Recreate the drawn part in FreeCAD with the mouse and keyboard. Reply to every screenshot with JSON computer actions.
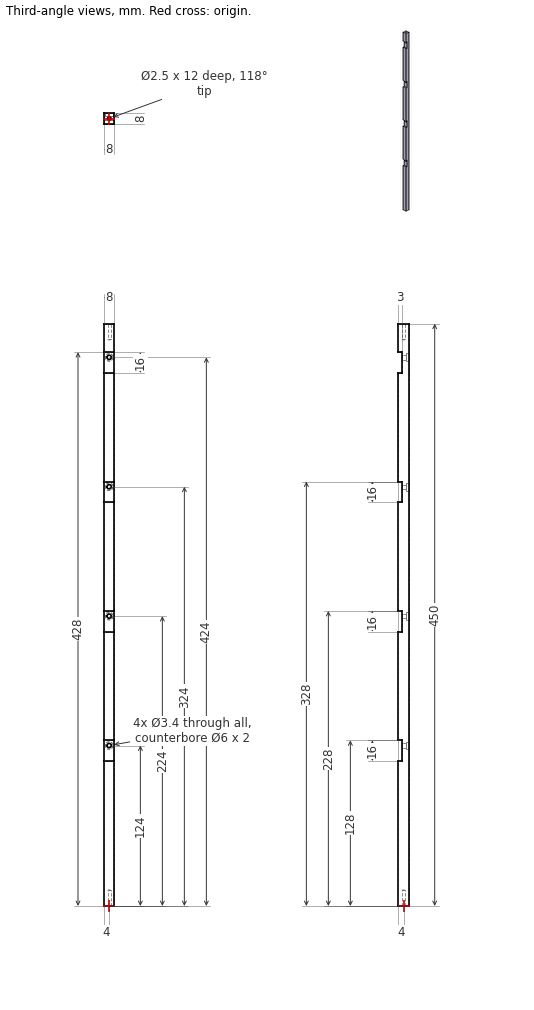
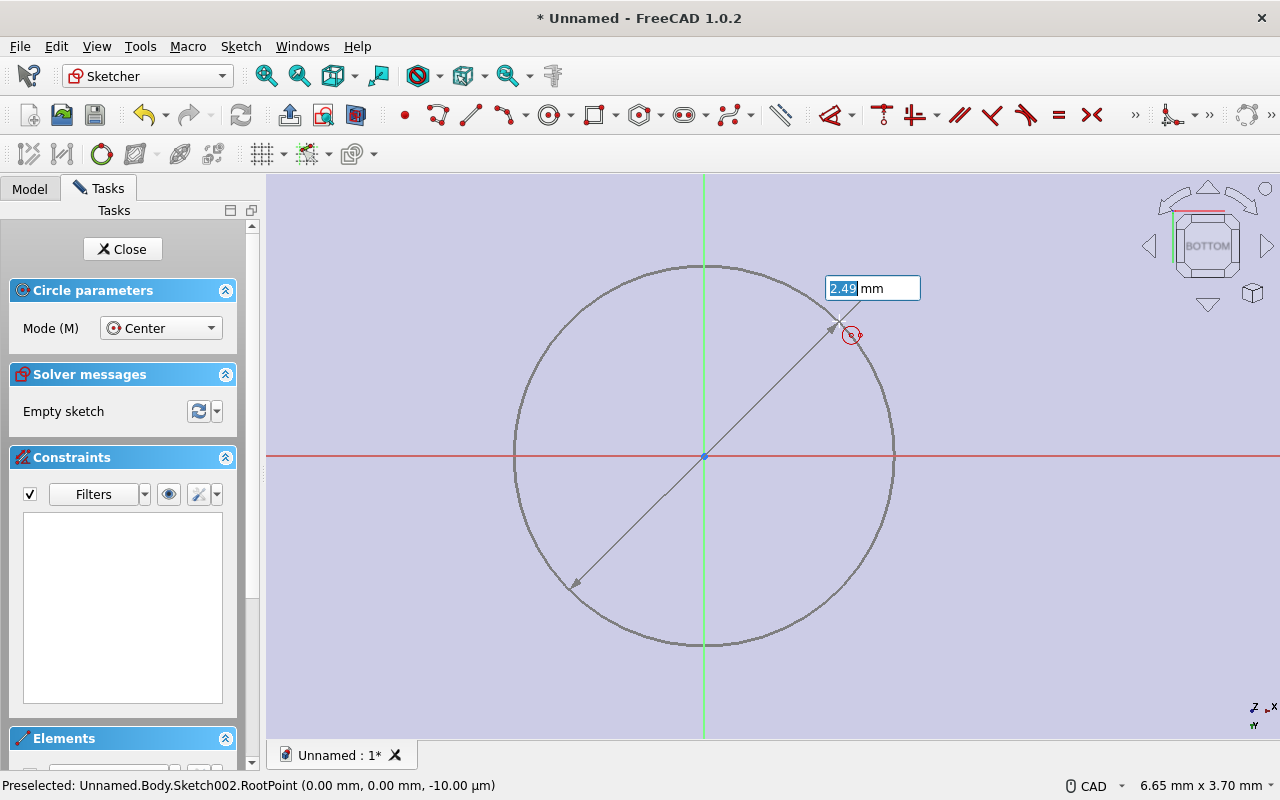
{"action": "type", "text": "2.5"}
{"action": "key", "text": "Return"}
{"action": "key", "text": "Escape"}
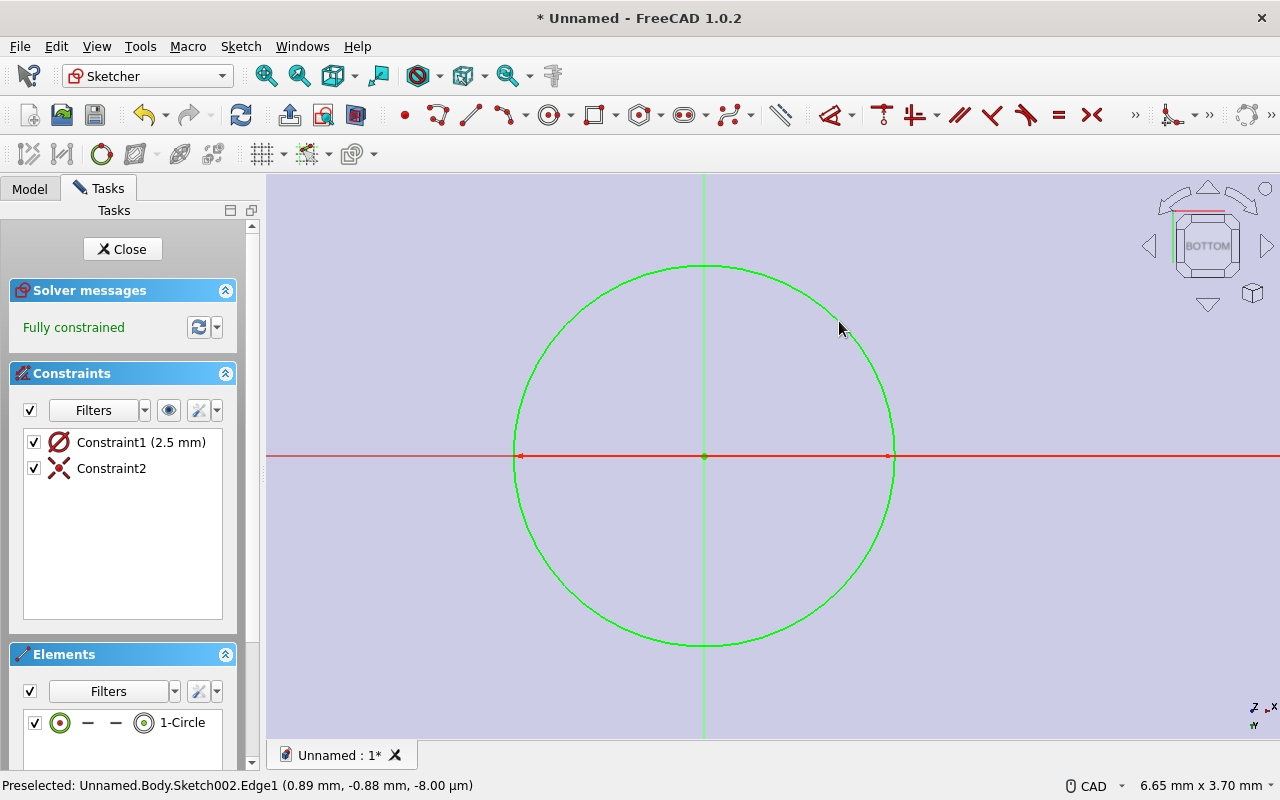
{"action": "left_click", "coordinate": [123, 249]}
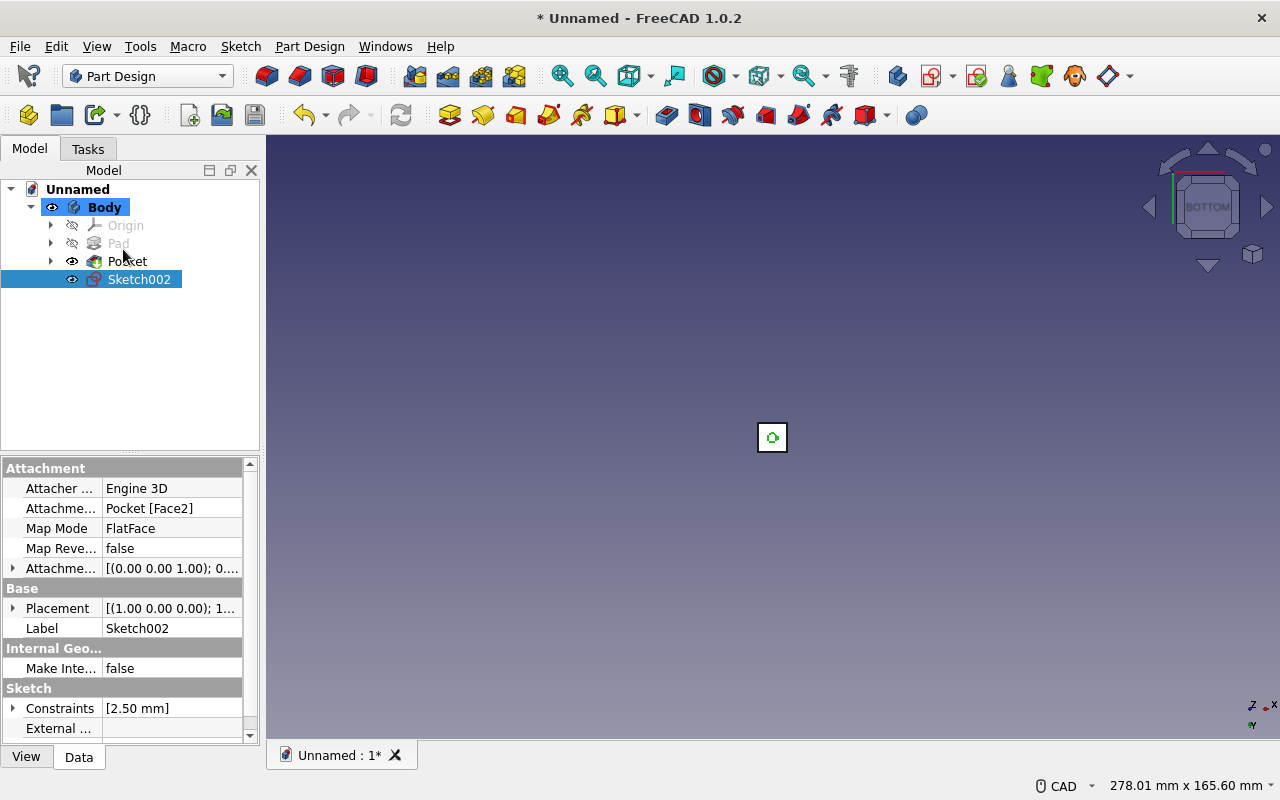
{"action": "left_click", "coordinate": [700, 116]}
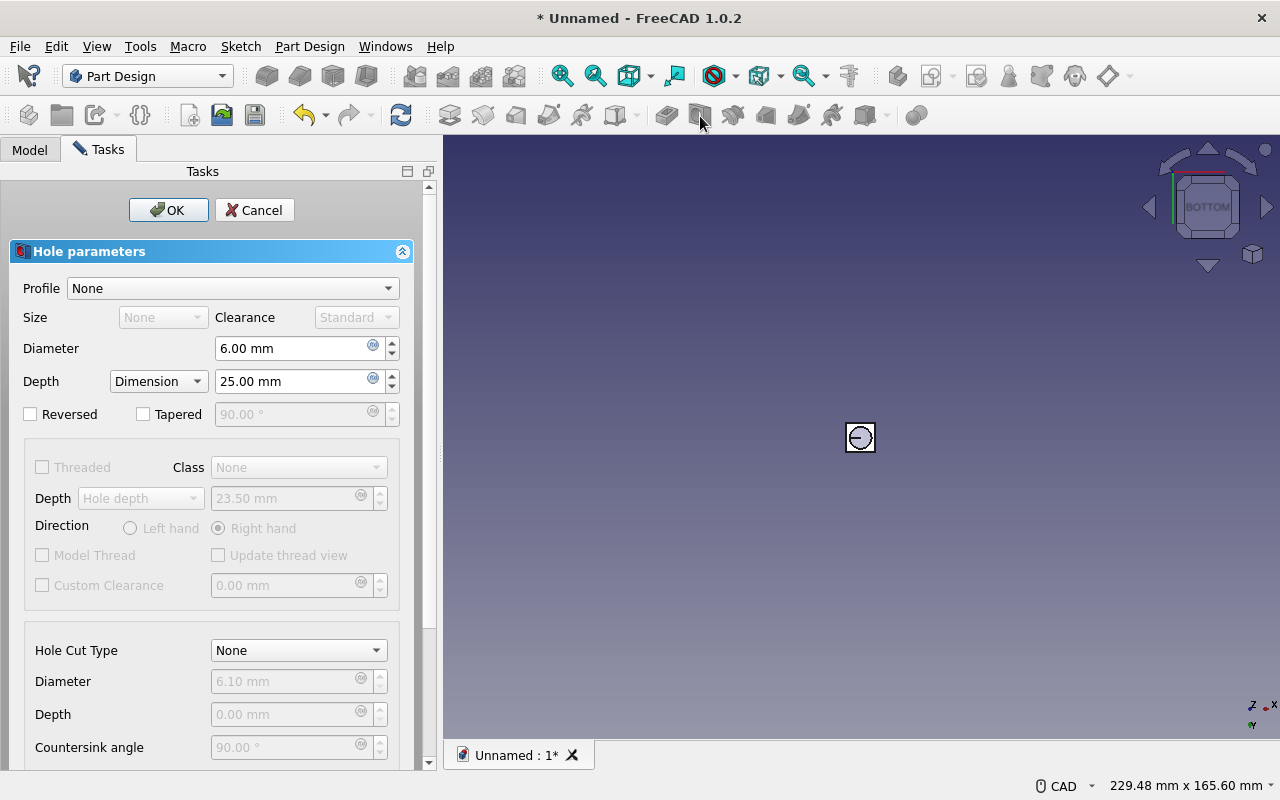
{"action": "triple_click", "coordinate": [300, 348]}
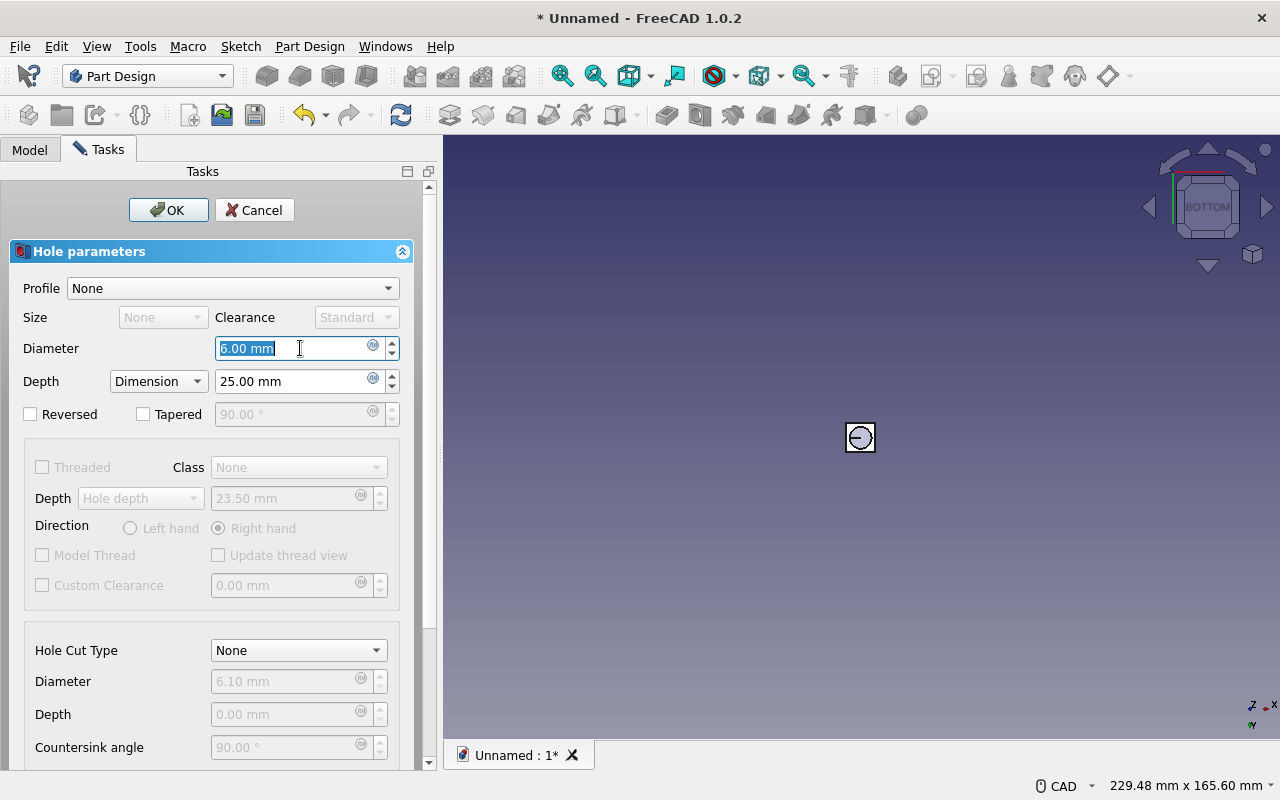
{"action": "type", "text": "2.5"}
{"action": "key", "text": "Tab"}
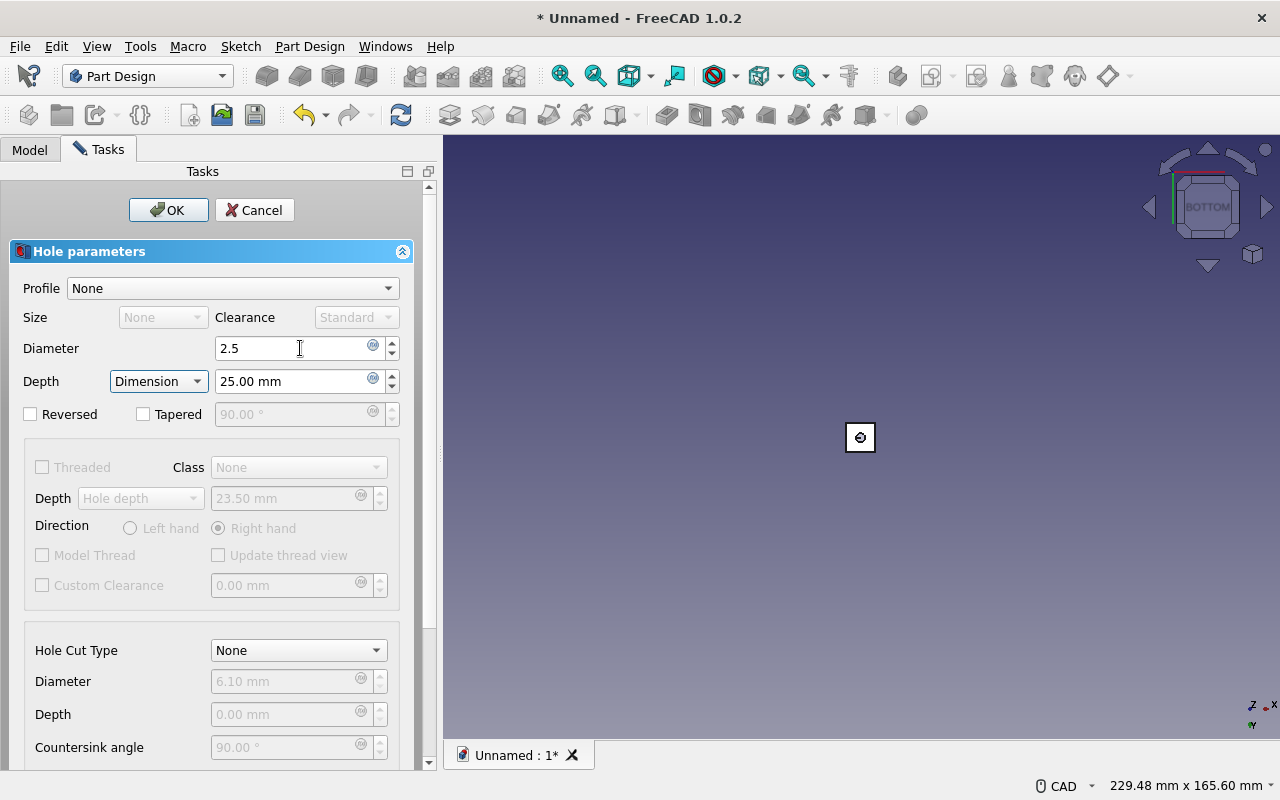
{"action": "triple_click", "coordinate": [300, 382]}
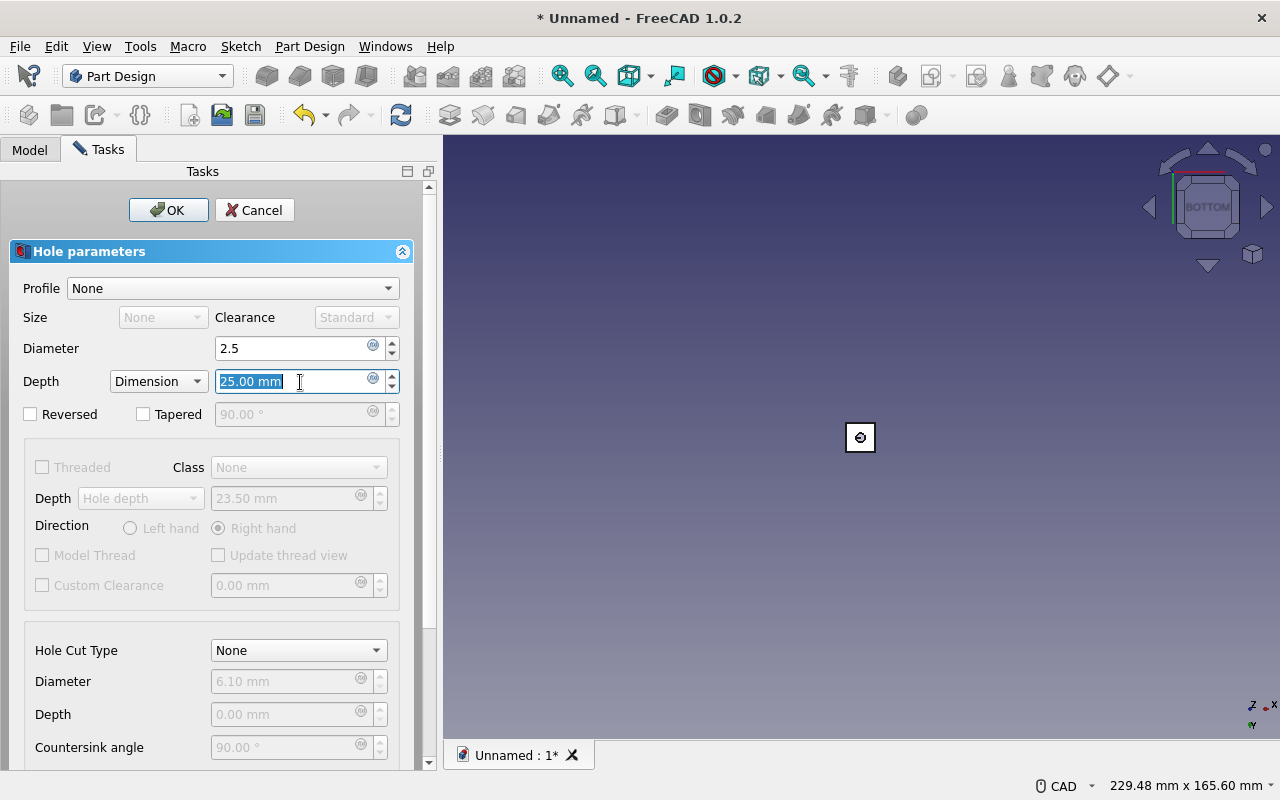
{"action": "type", "text": "12"}
{"action": "key", "text": "Tab"}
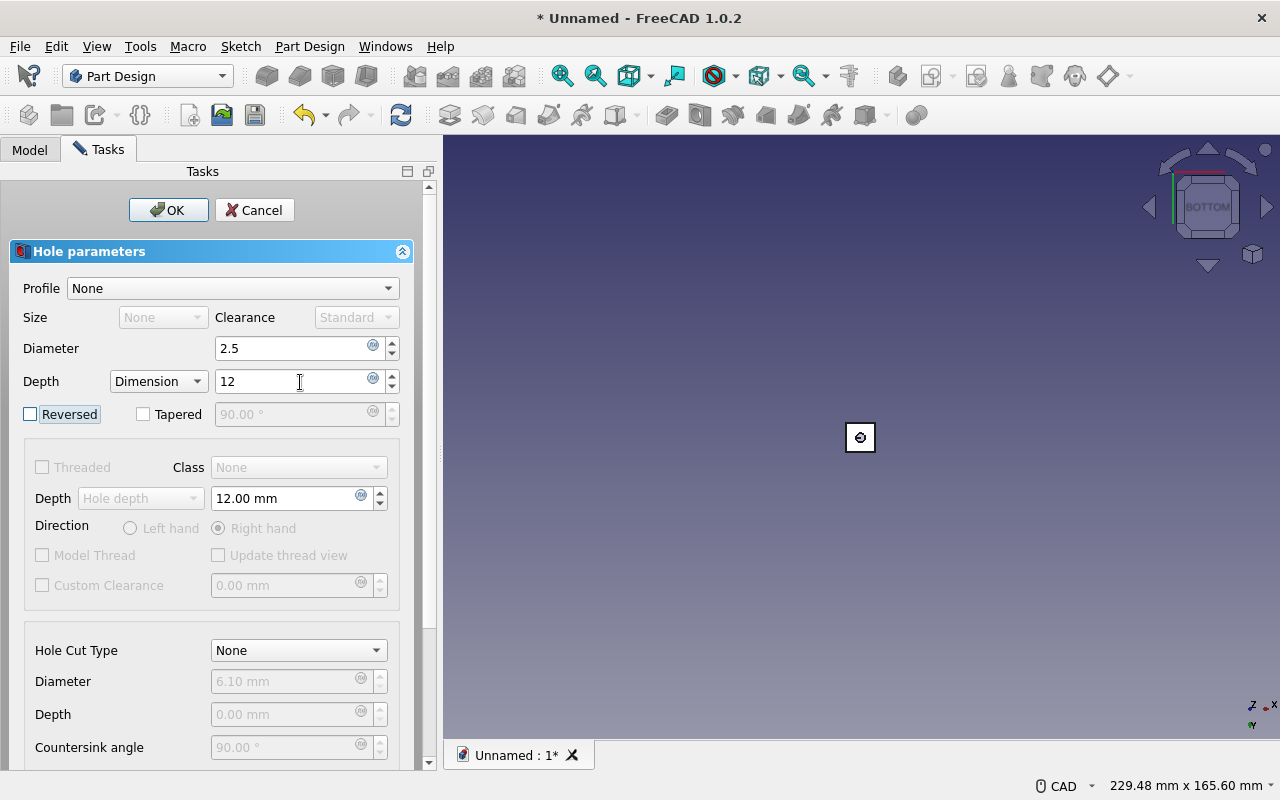
{"action": "left_click", "coordinate": [169, 210]}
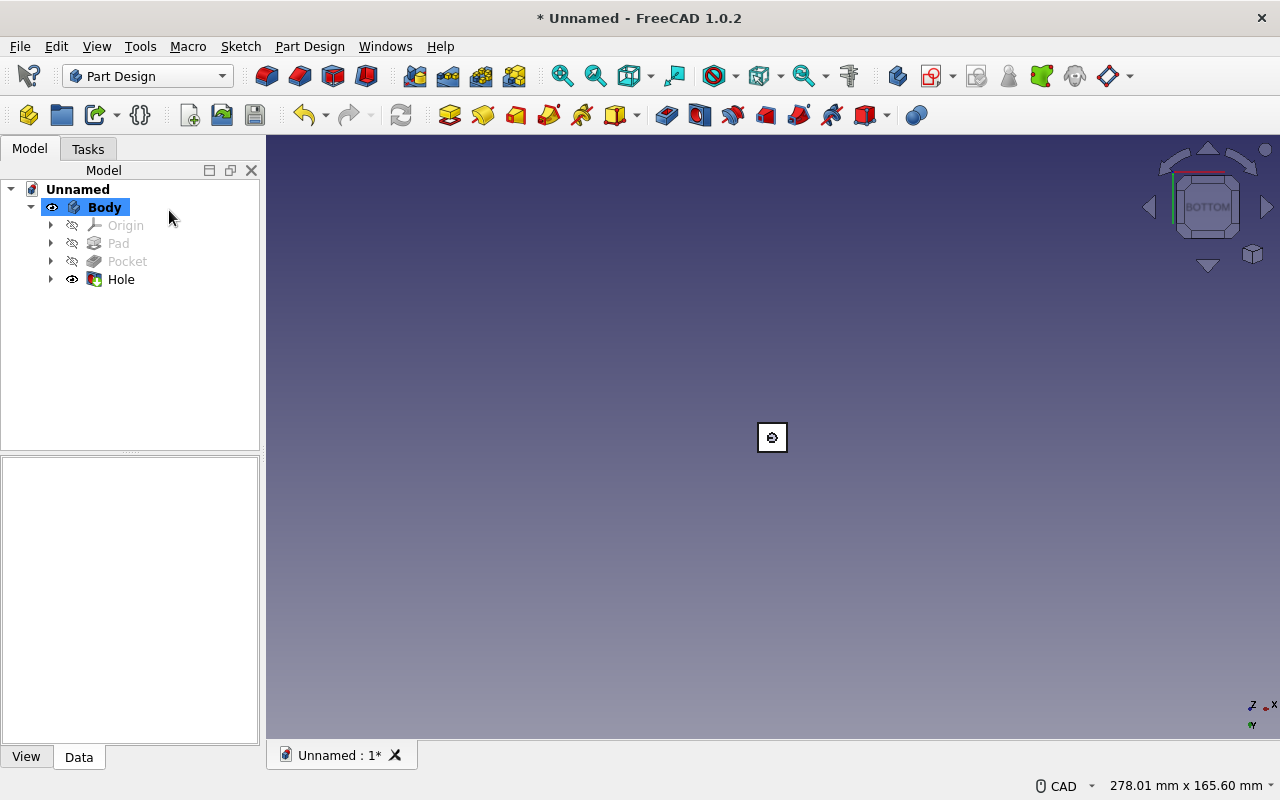
{"action": "key", "text": "v f"}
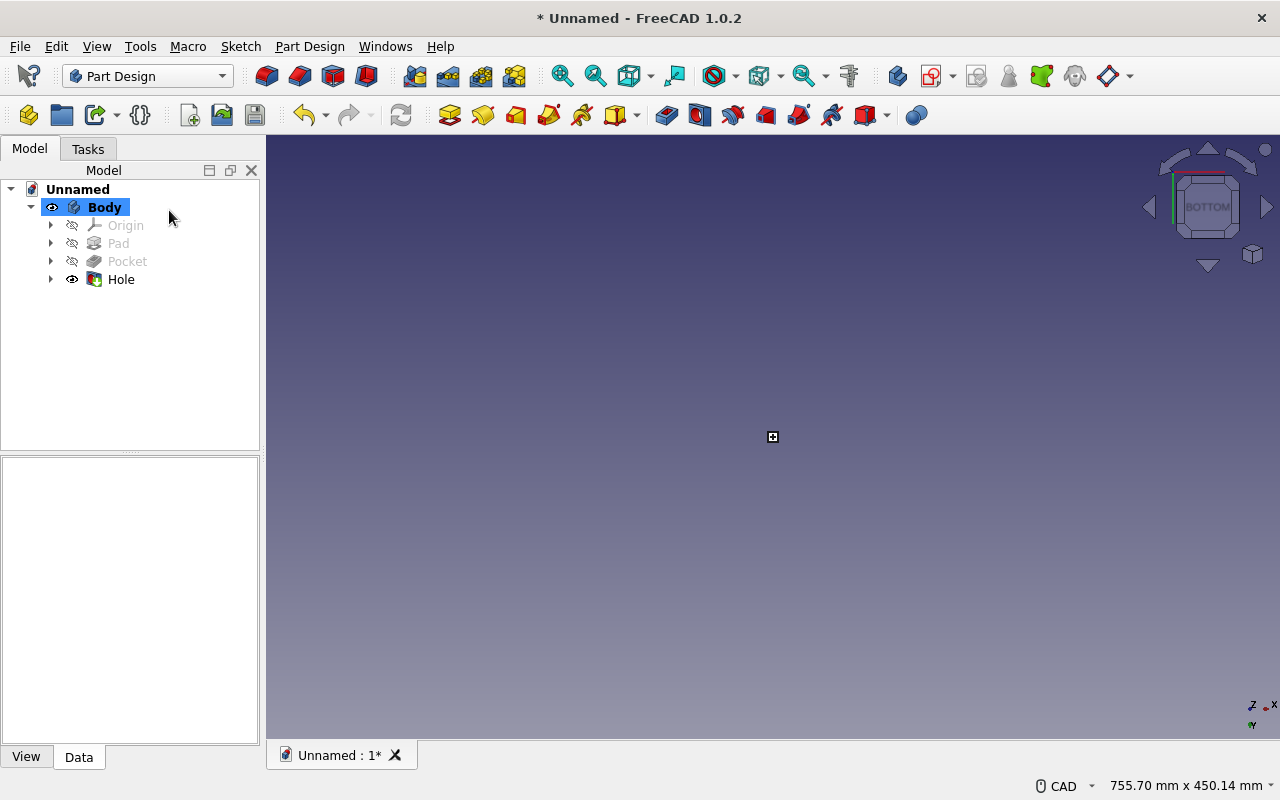
{"action": "key", "text": "0"}